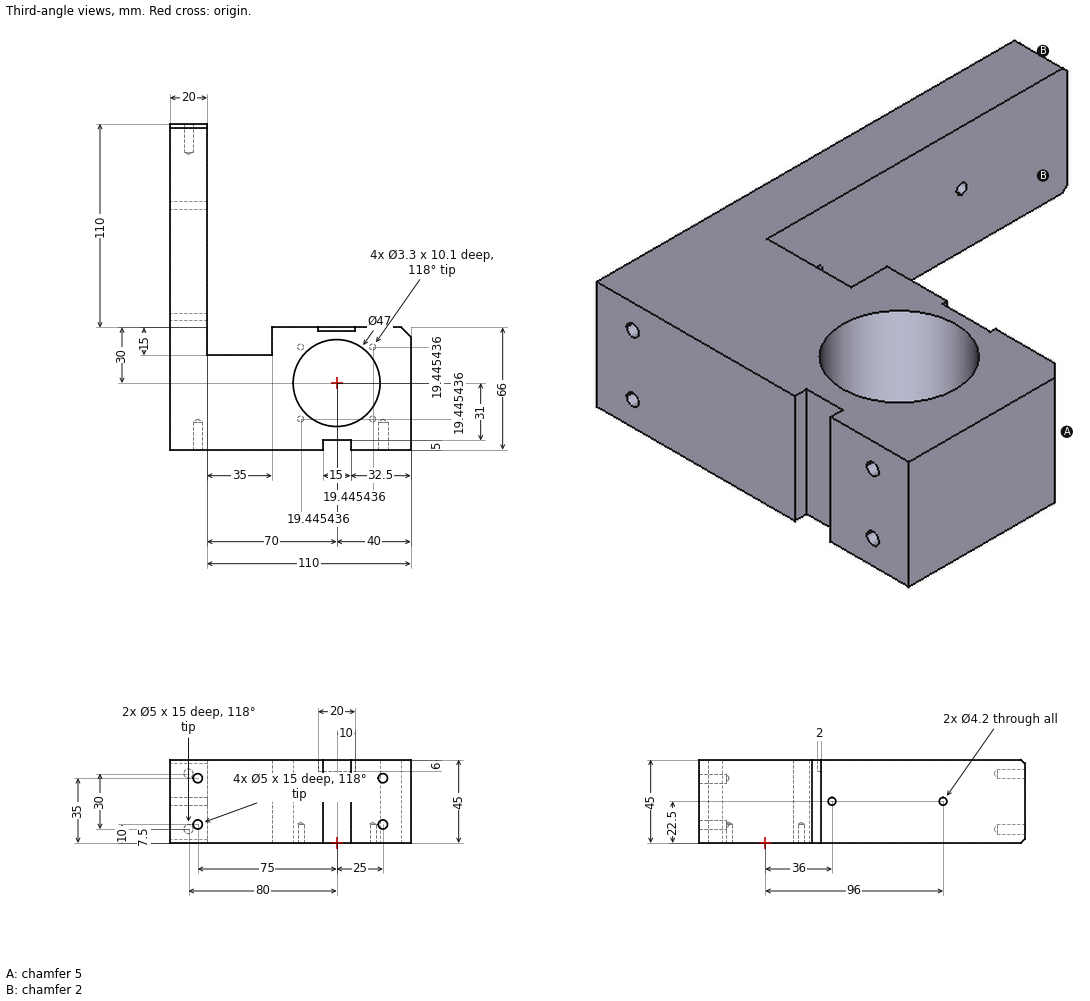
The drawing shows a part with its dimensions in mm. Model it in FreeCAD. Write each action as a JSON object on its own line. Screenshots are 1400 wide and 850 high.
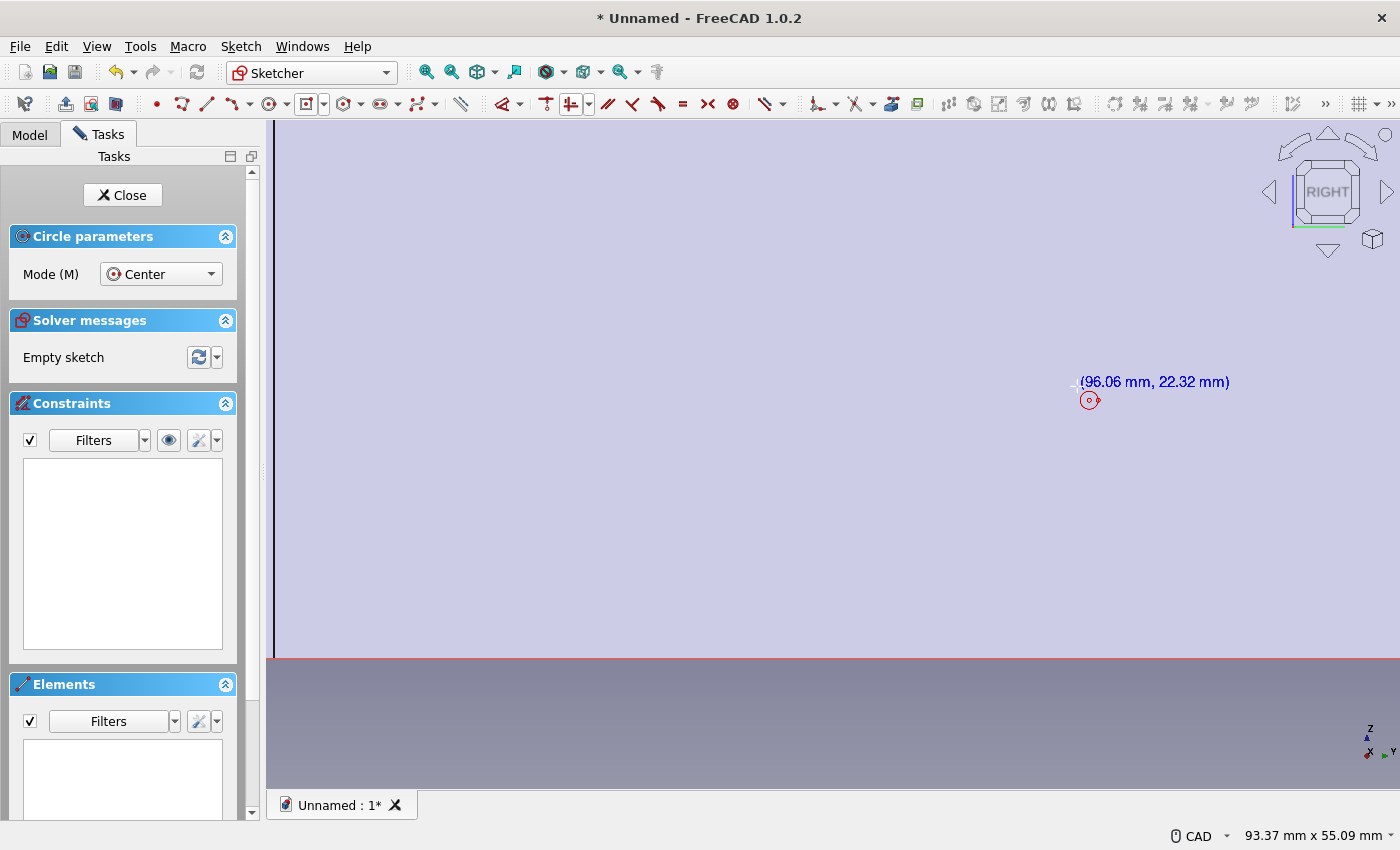
{"action": "left_click", "coordinate": [1076, 385]}
{"action": "left_click", "coordinate": [1094, 367]}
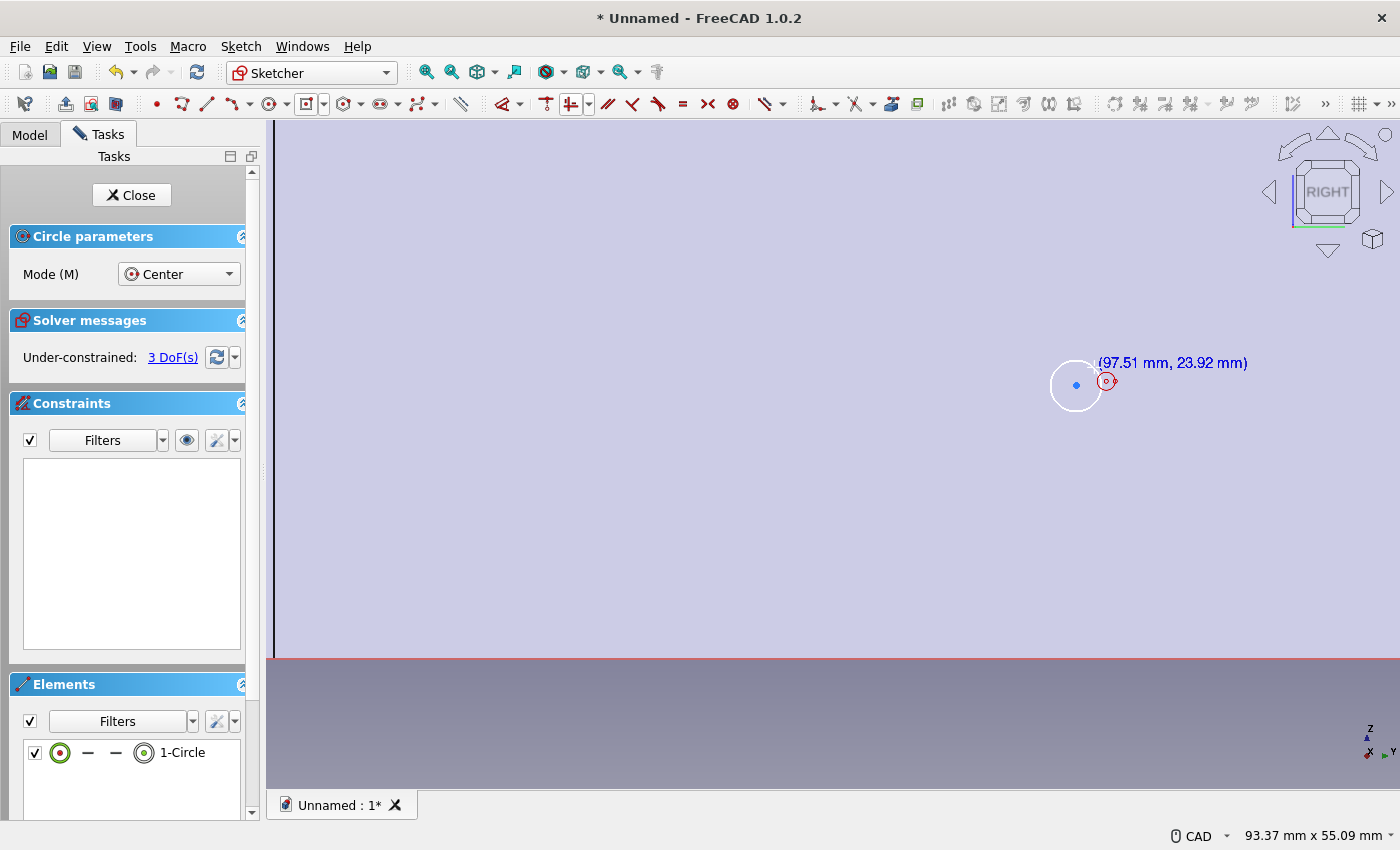
{"action": "left_click", "coordinate": [347, 385]}
{"action": "left_click", "coordinate": [365, 367]}
{"action": "key", "text": "Escape"}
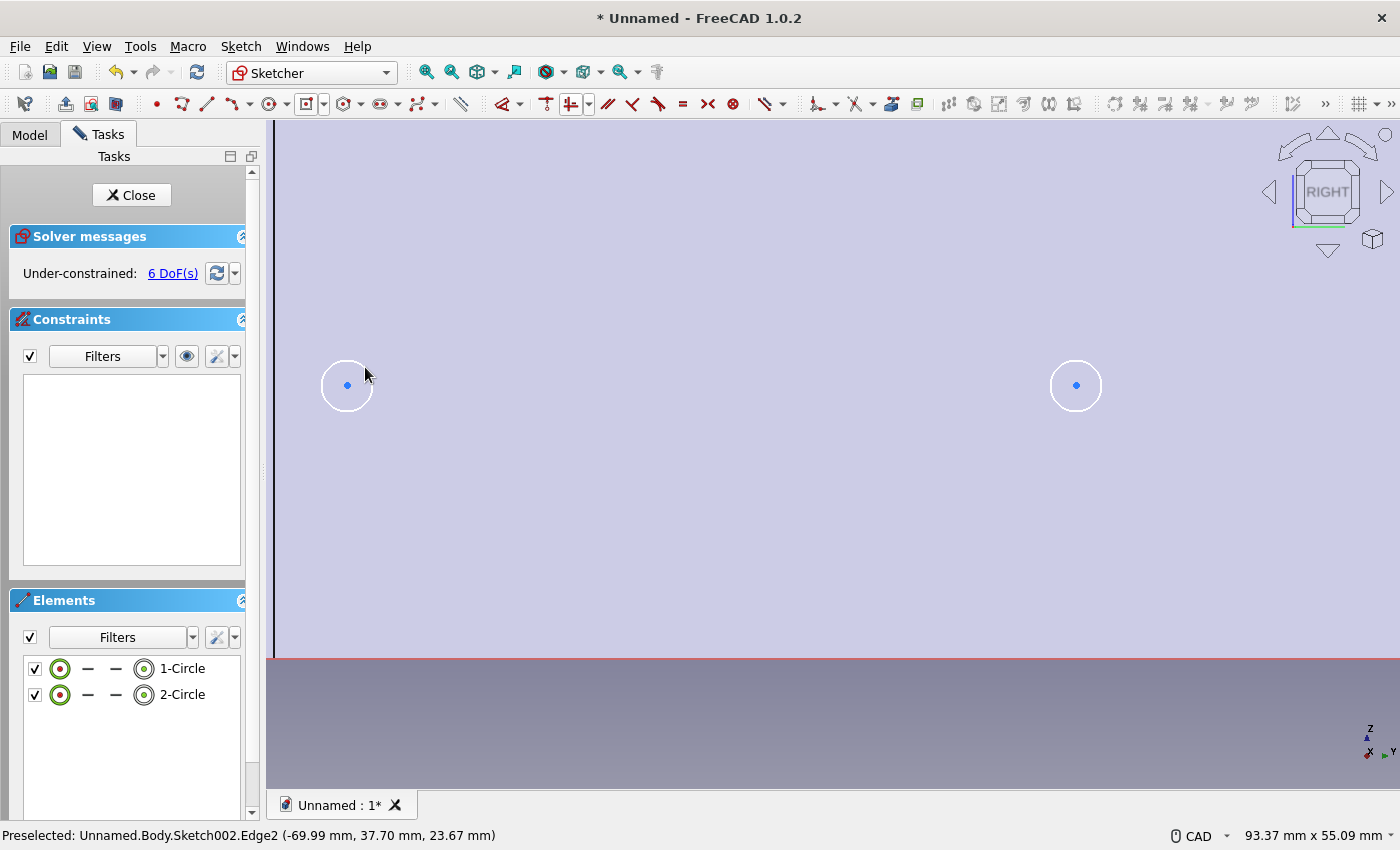
{"action": "left_click", "coordinate": [1094, 368]}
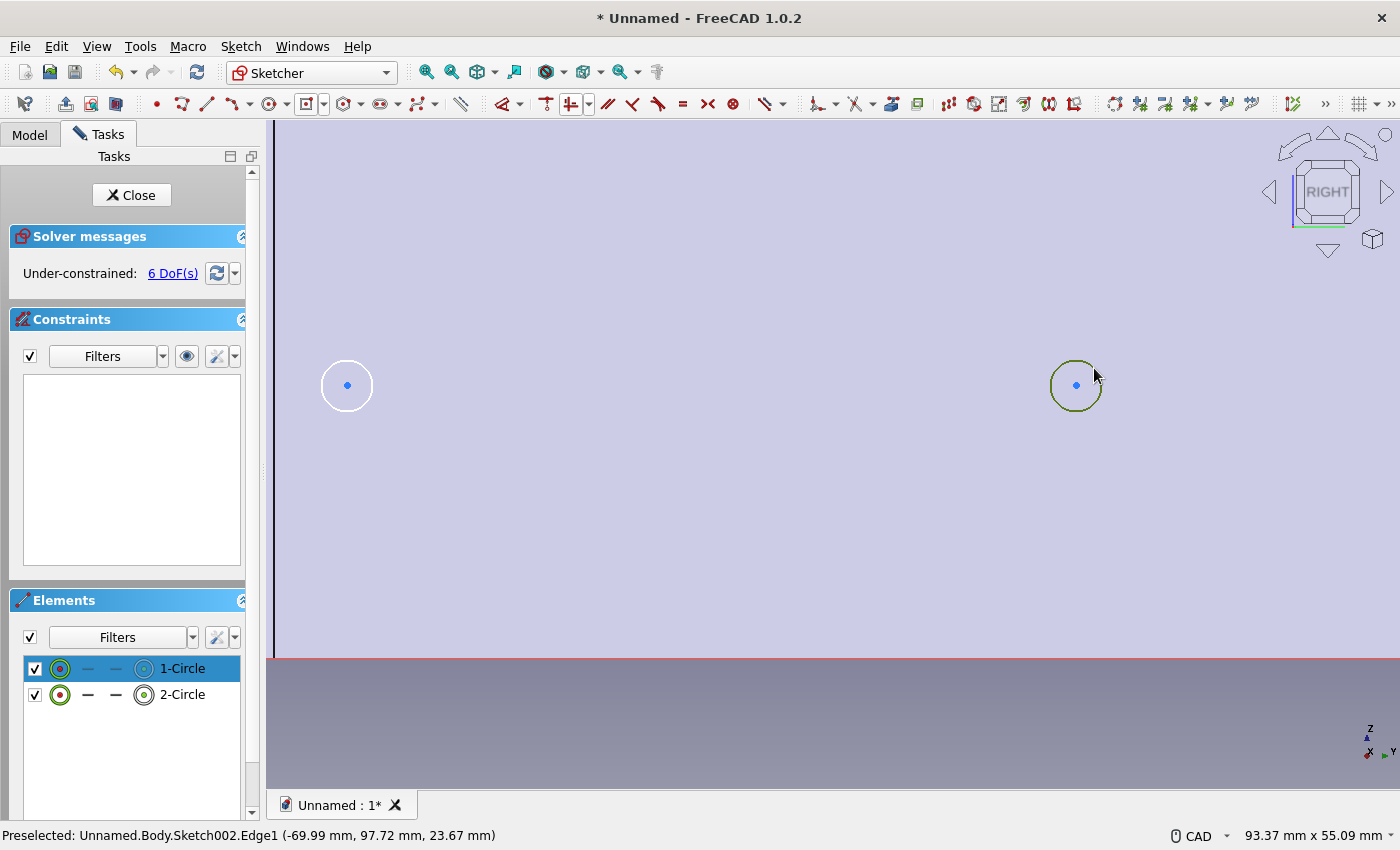
{"action": "left_click", "coordinate": [365, 368]}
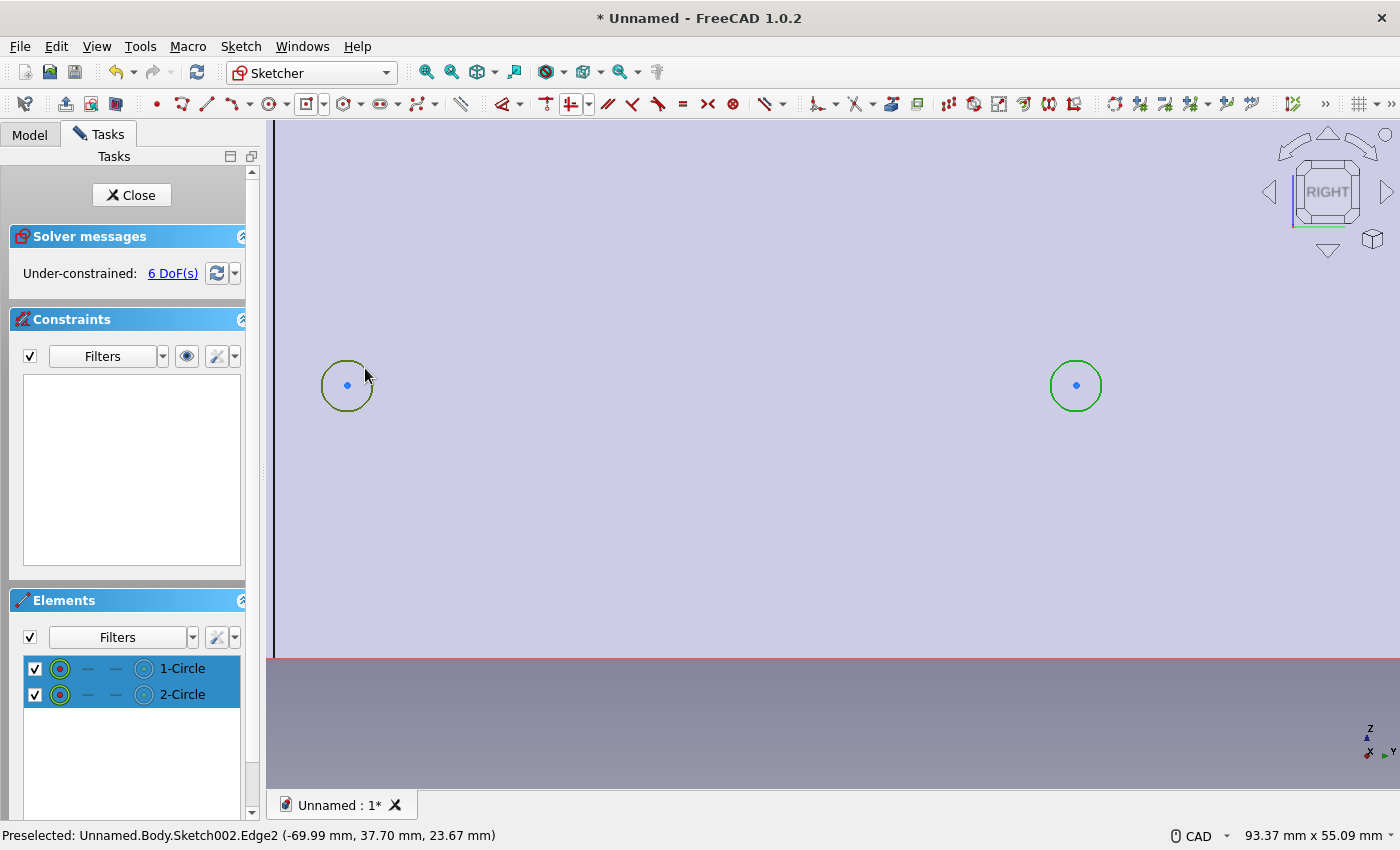
{"action": "left_click", "coordinate": [683, 104]}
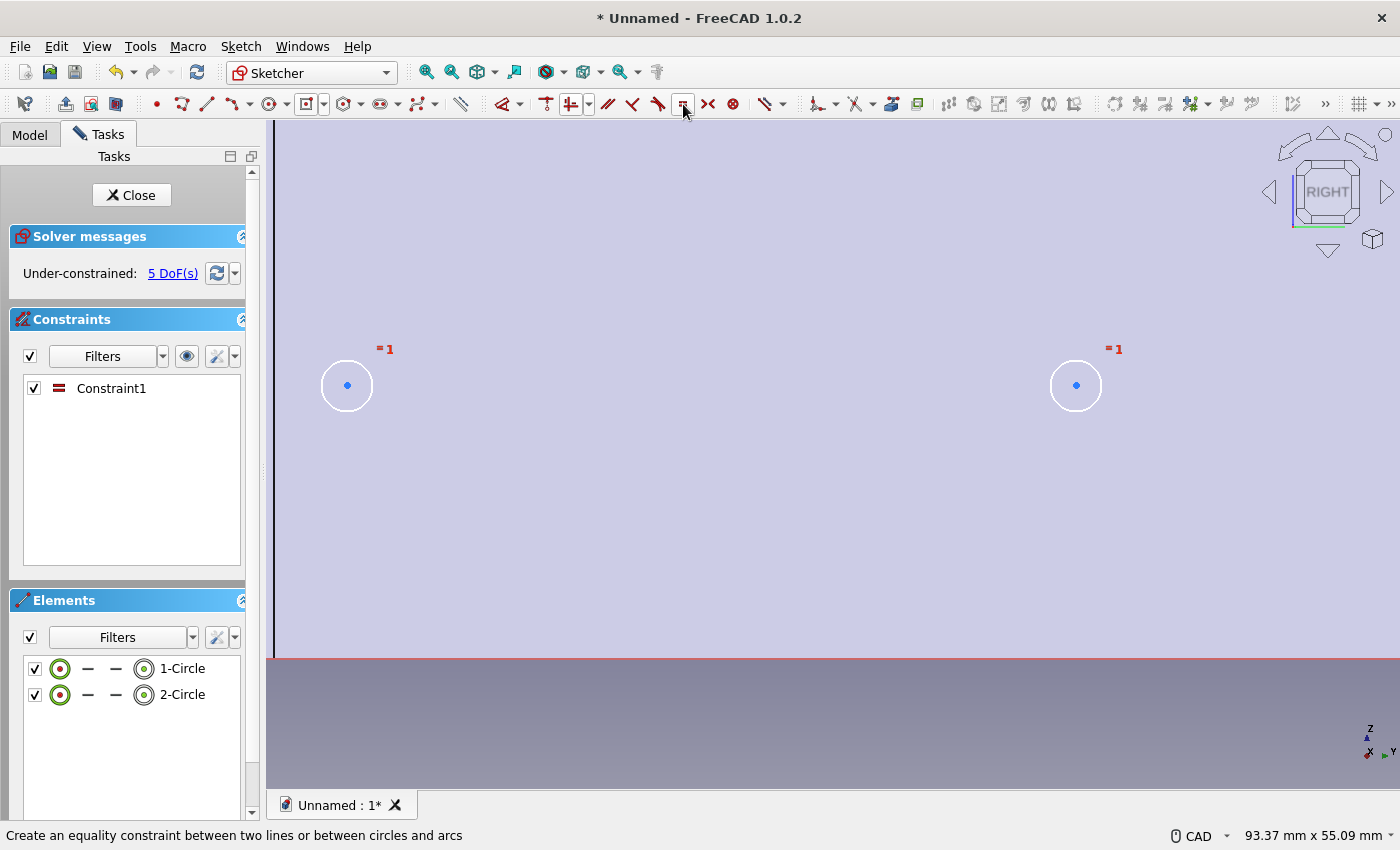
{"action": "left_click", "coordinate": [1076, 386]}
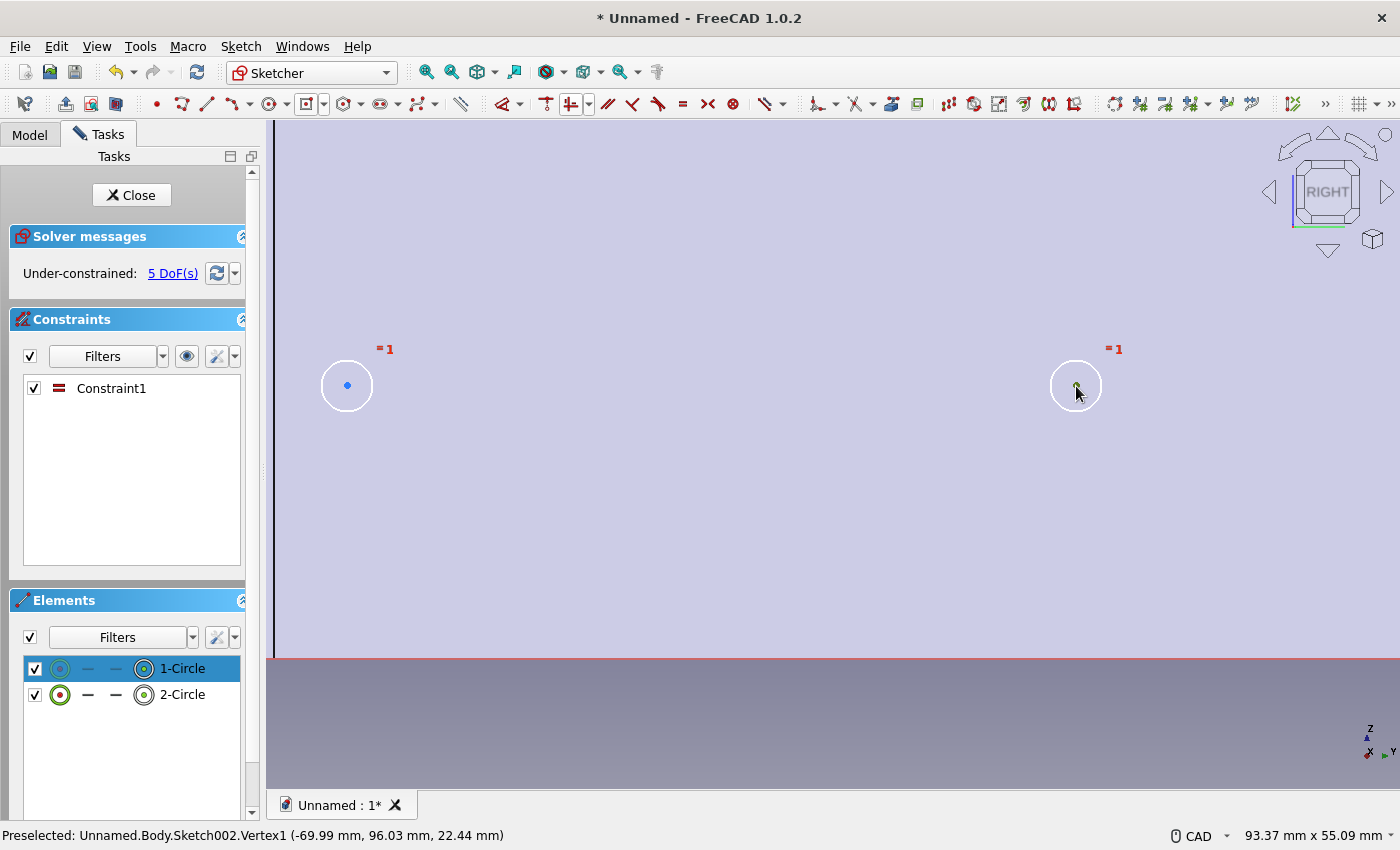
{"action": "left_click", "coordinate": [347, 386]}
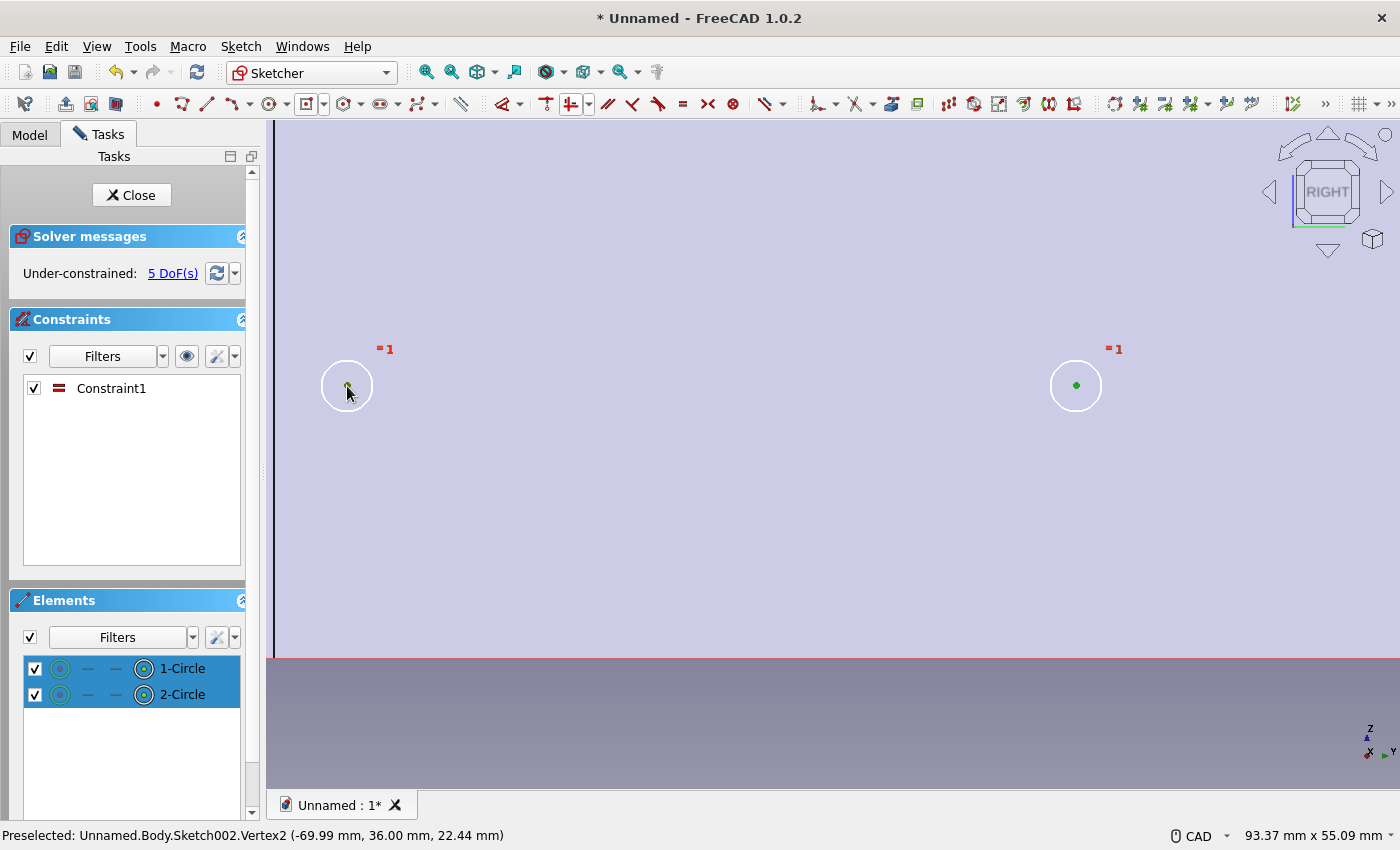
{"action": "key", "text": "h"}